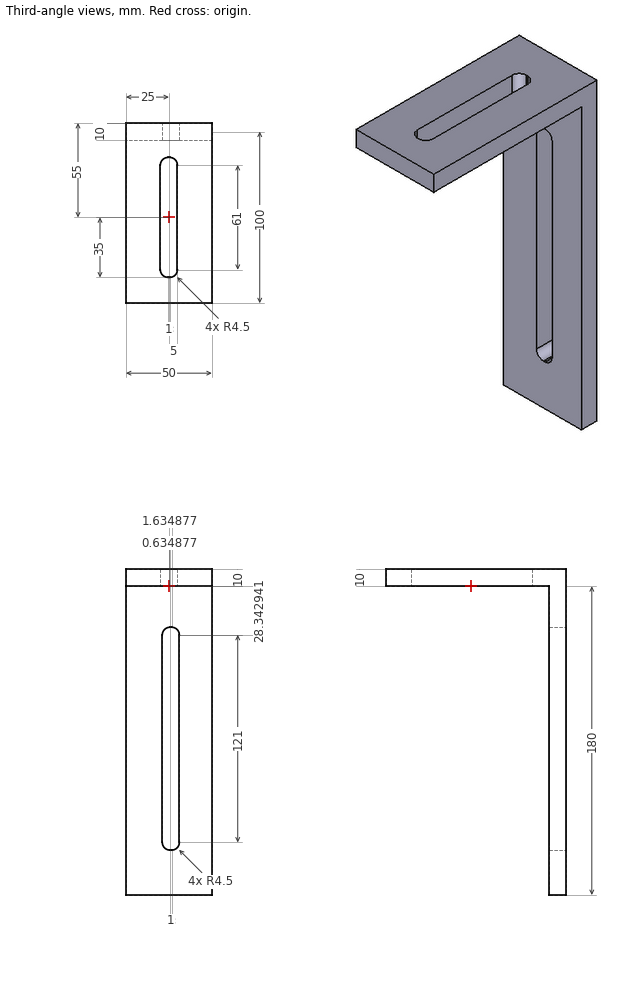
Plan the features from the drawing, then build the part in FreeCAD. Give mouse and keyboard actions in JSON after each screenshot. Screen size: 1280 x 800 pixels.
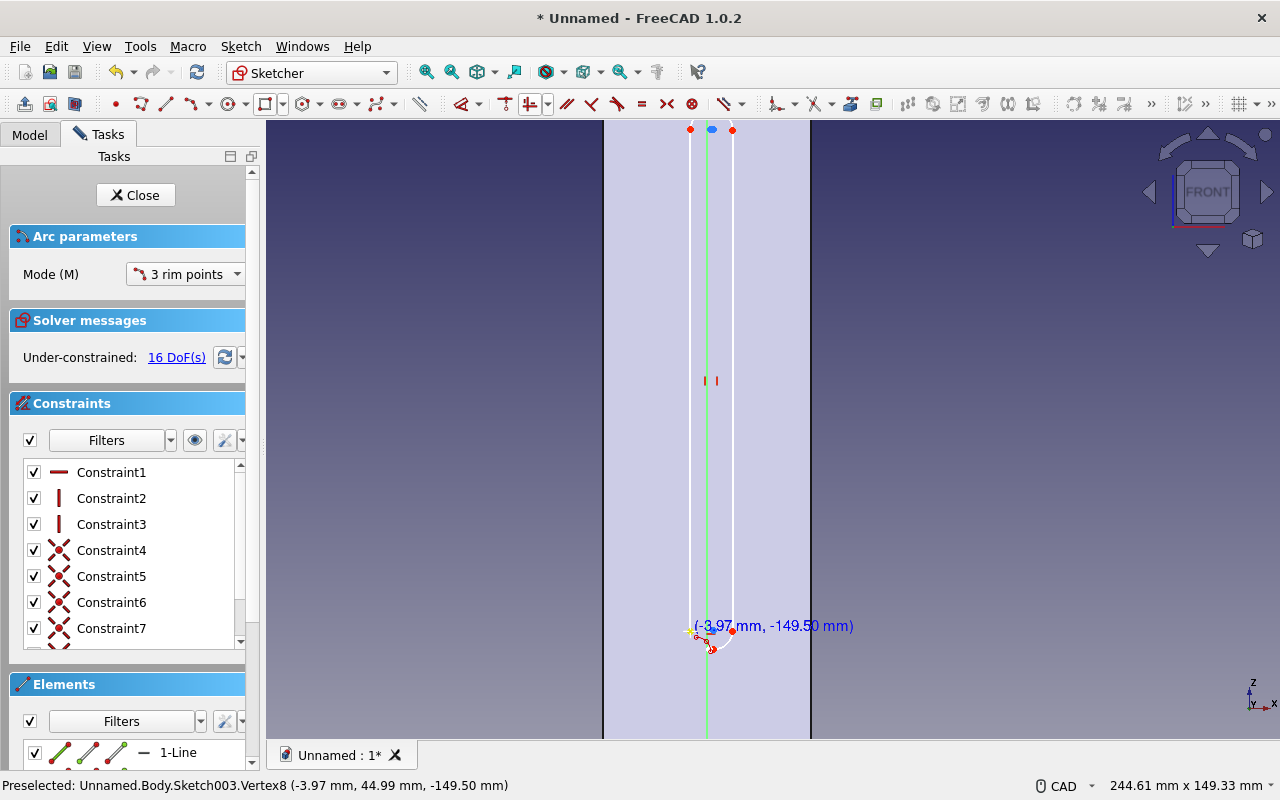
{"action": "scroll", "coordinate": [710, 649], "scroll_direction": "up", "scroll_amount": 11}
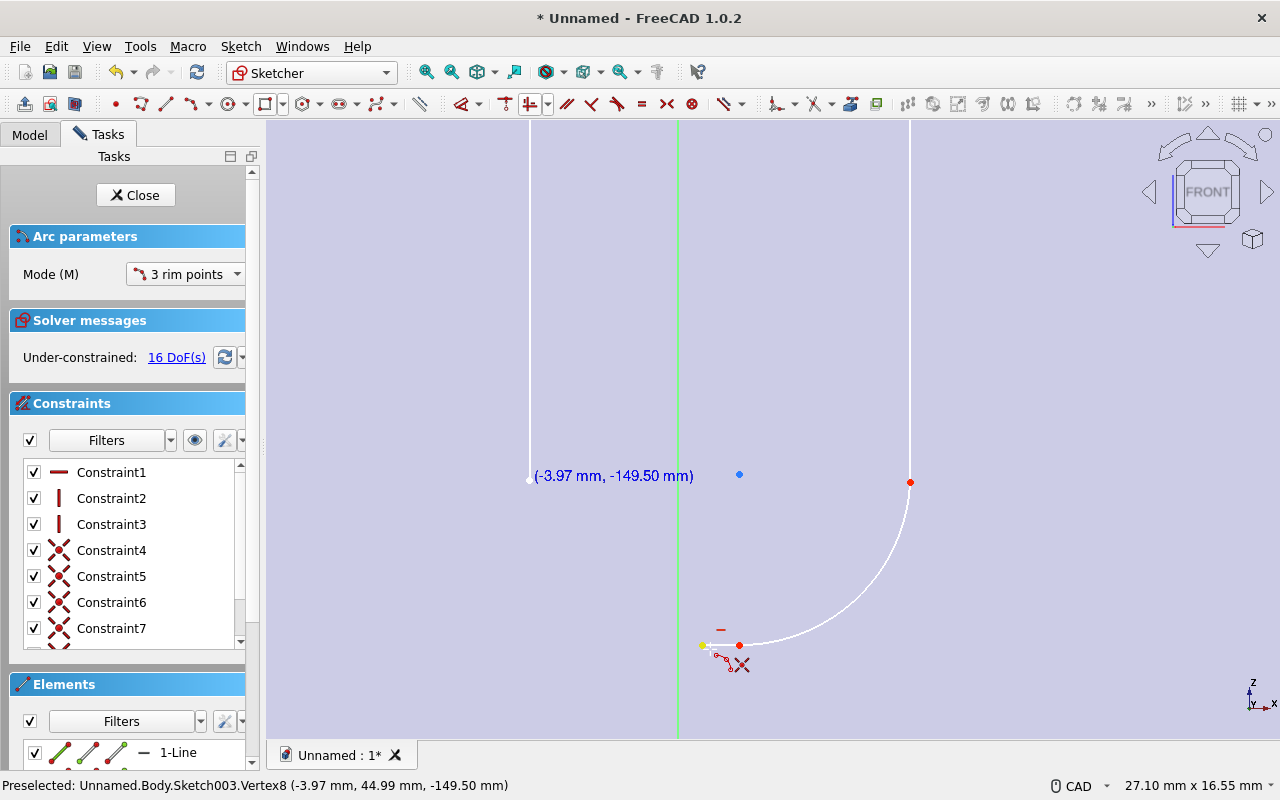
{"action": "left_click", "coordinate": [702, 645]}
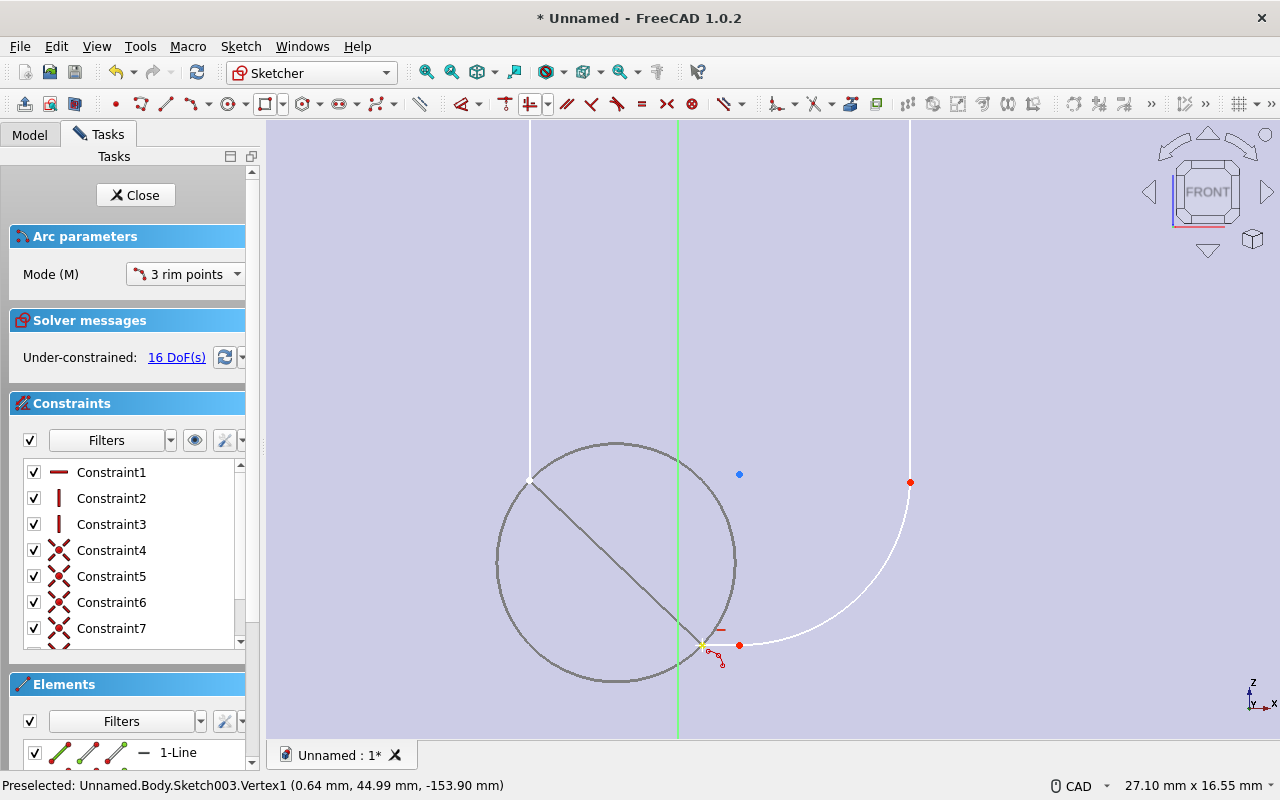
{"action": "scroll", "coordinate": [703, 643], "scroll_direction": "down", "scroll_amount": 13}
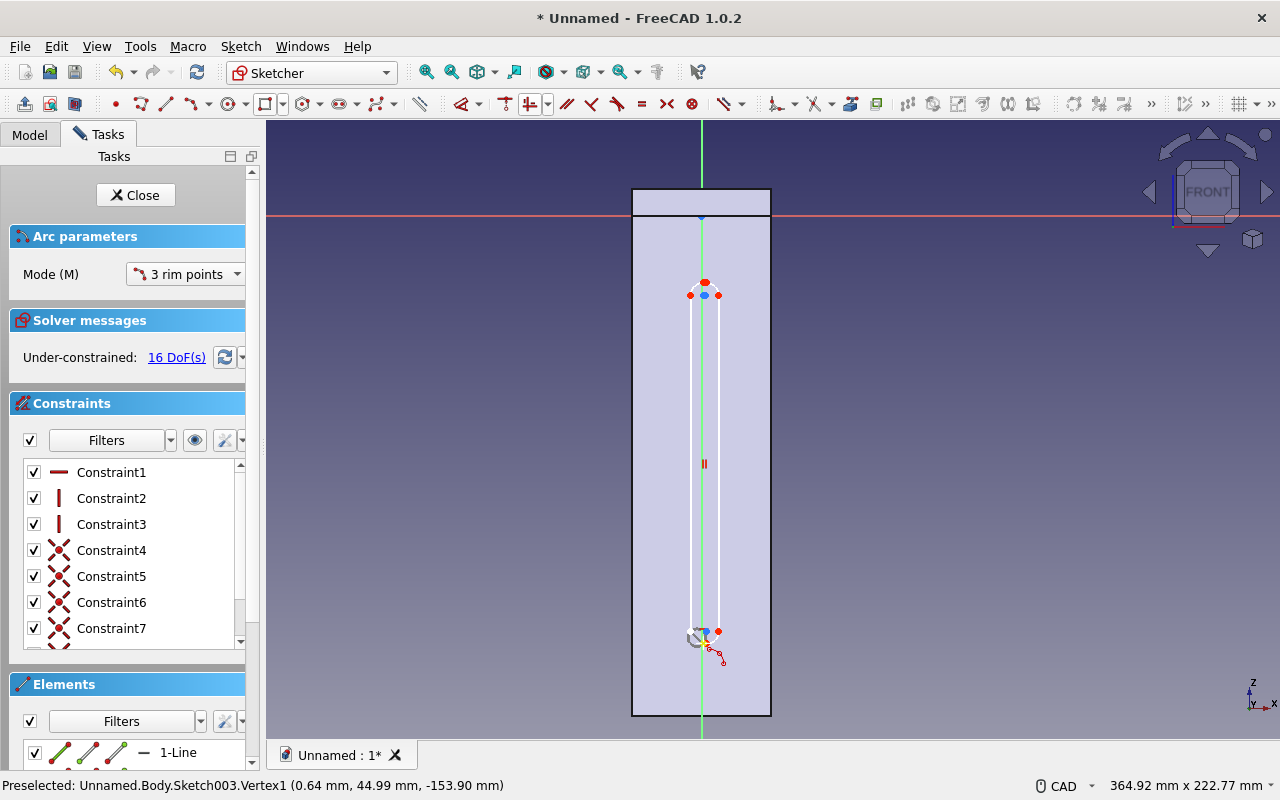
{"action": "scroll", "coordinate": [694, 640], "scroll_direction": "up", "scroll_amount": 8}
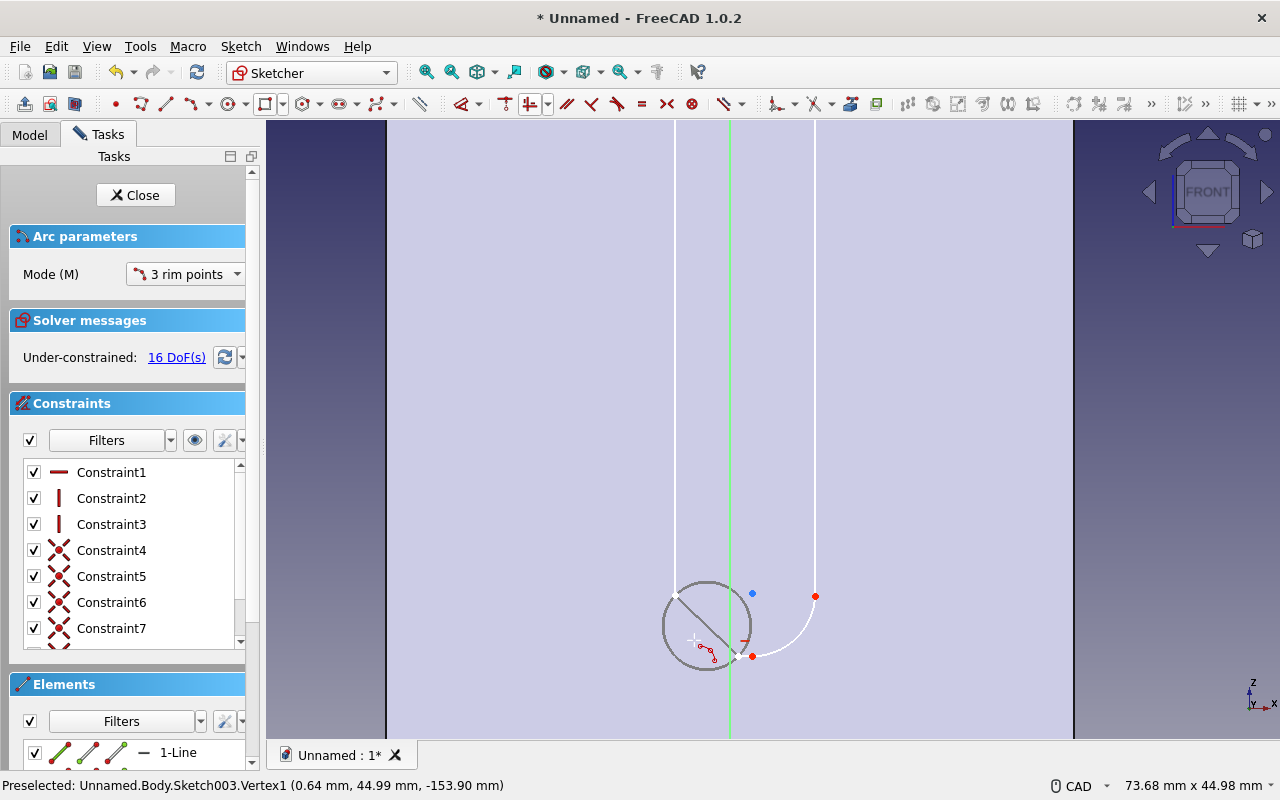
{"action": "left_click", "coordinate": [695, 637]}
{"action": "key", "text": "Escape"}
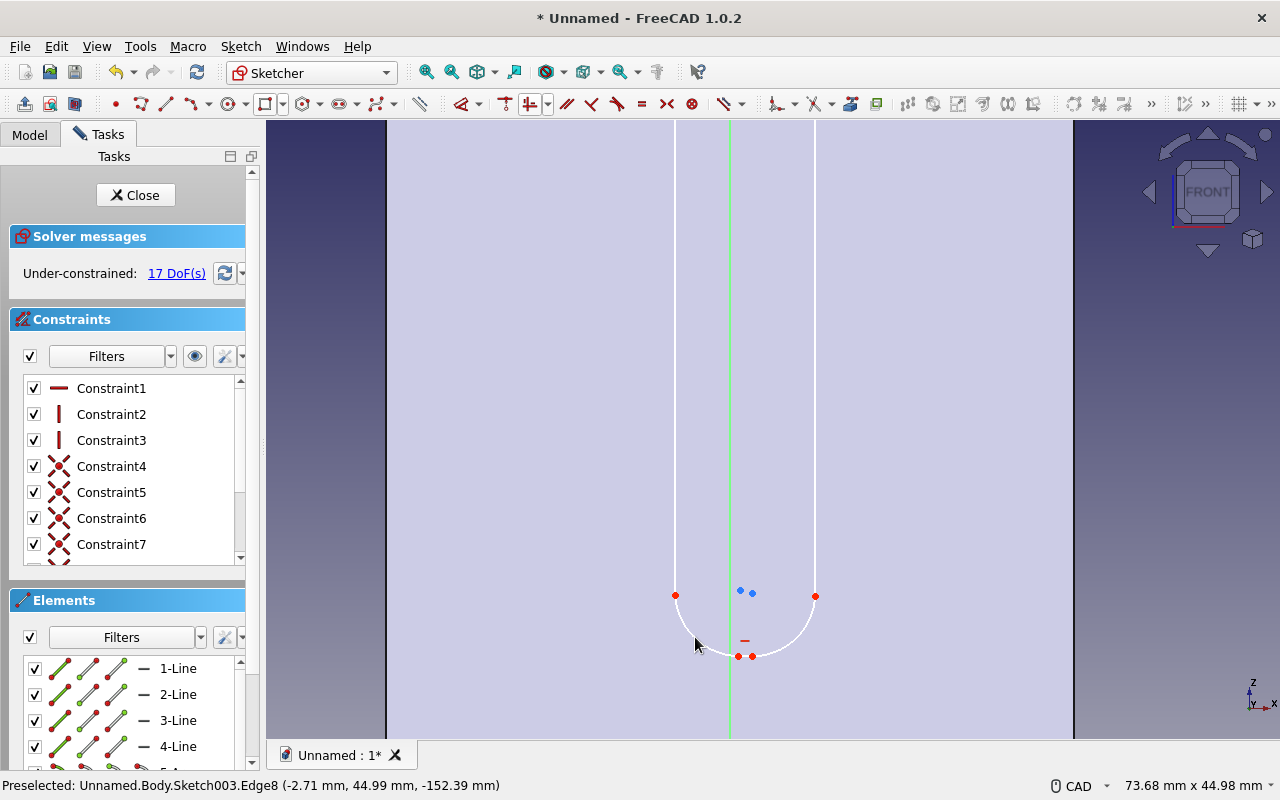
{"action": "scroll", "coordinate": [746, 656], "scroll_direction": "up", "scroll_amount": 4}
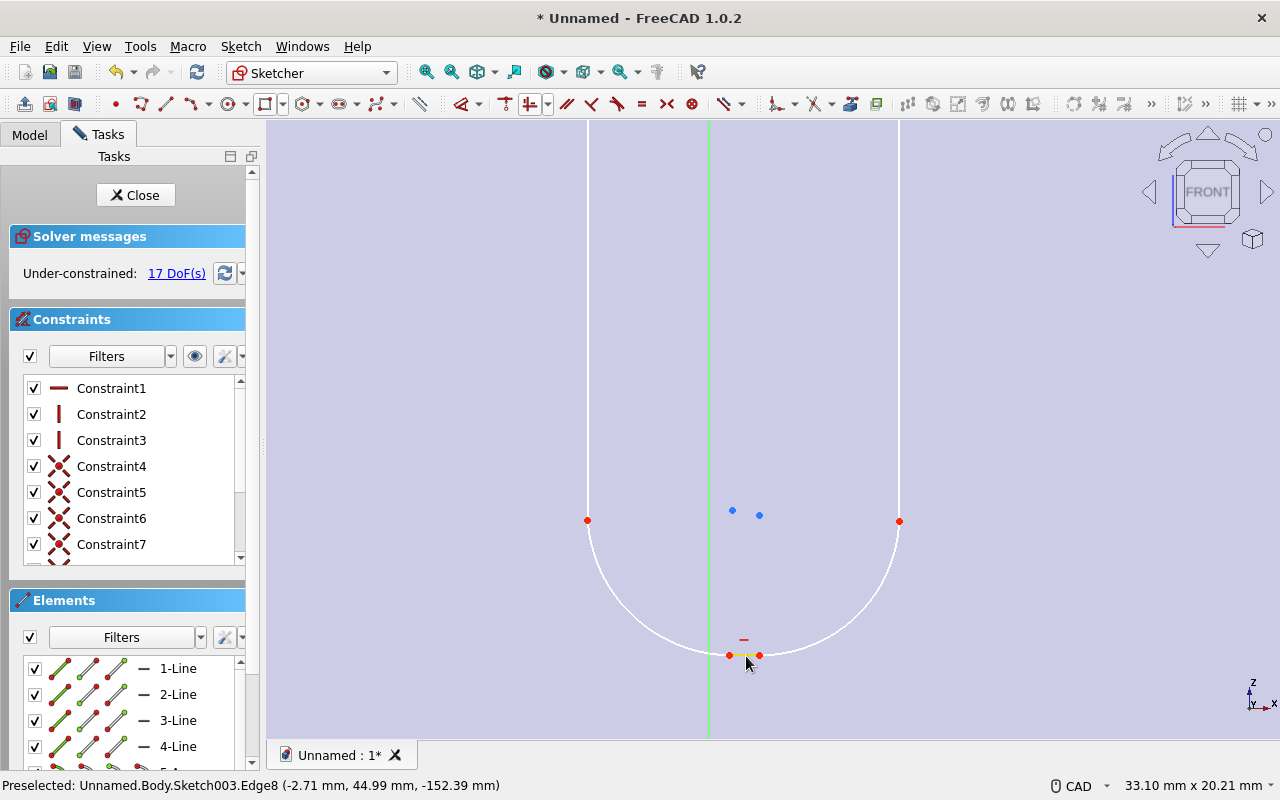
{"action": "left_click", "coordinate": [744, 655]}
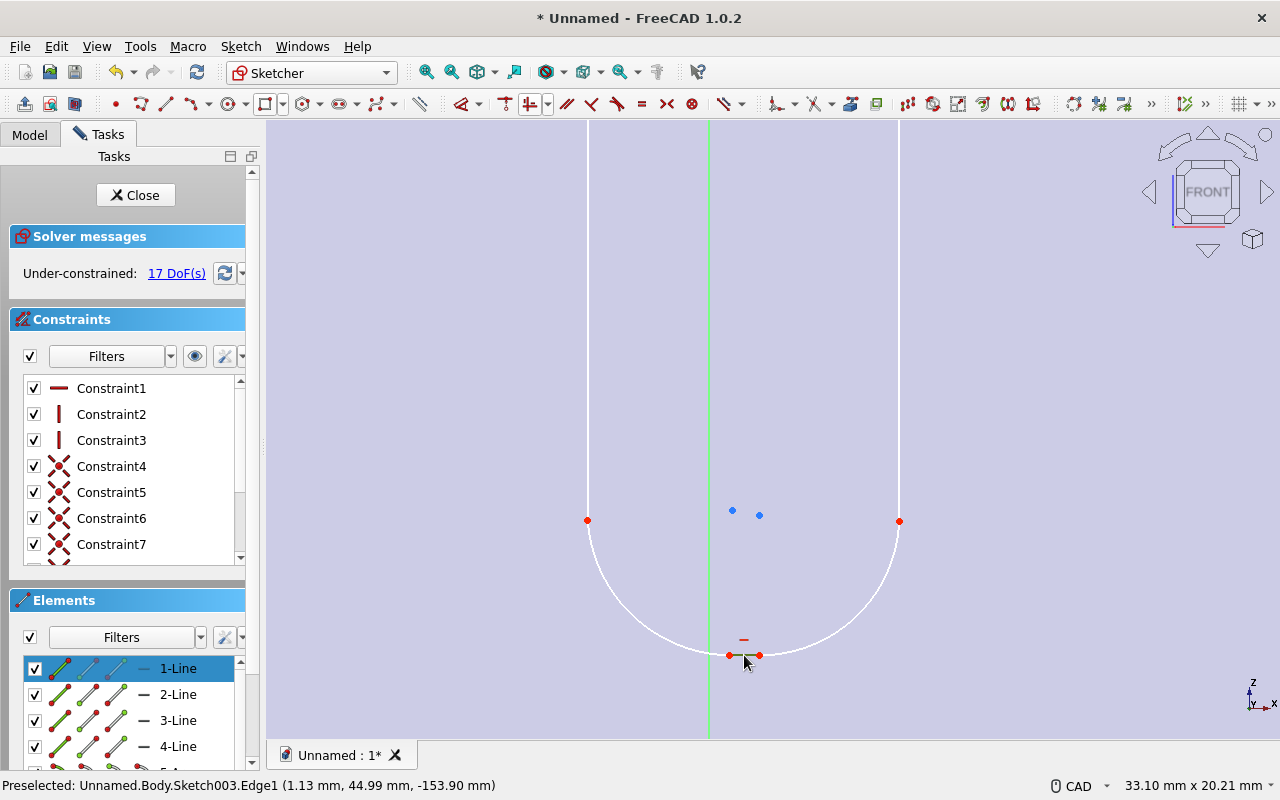
{"action": "scroll", "coordinate": [701, 642], "scroll_direction": "down", "scroll_amount": 12}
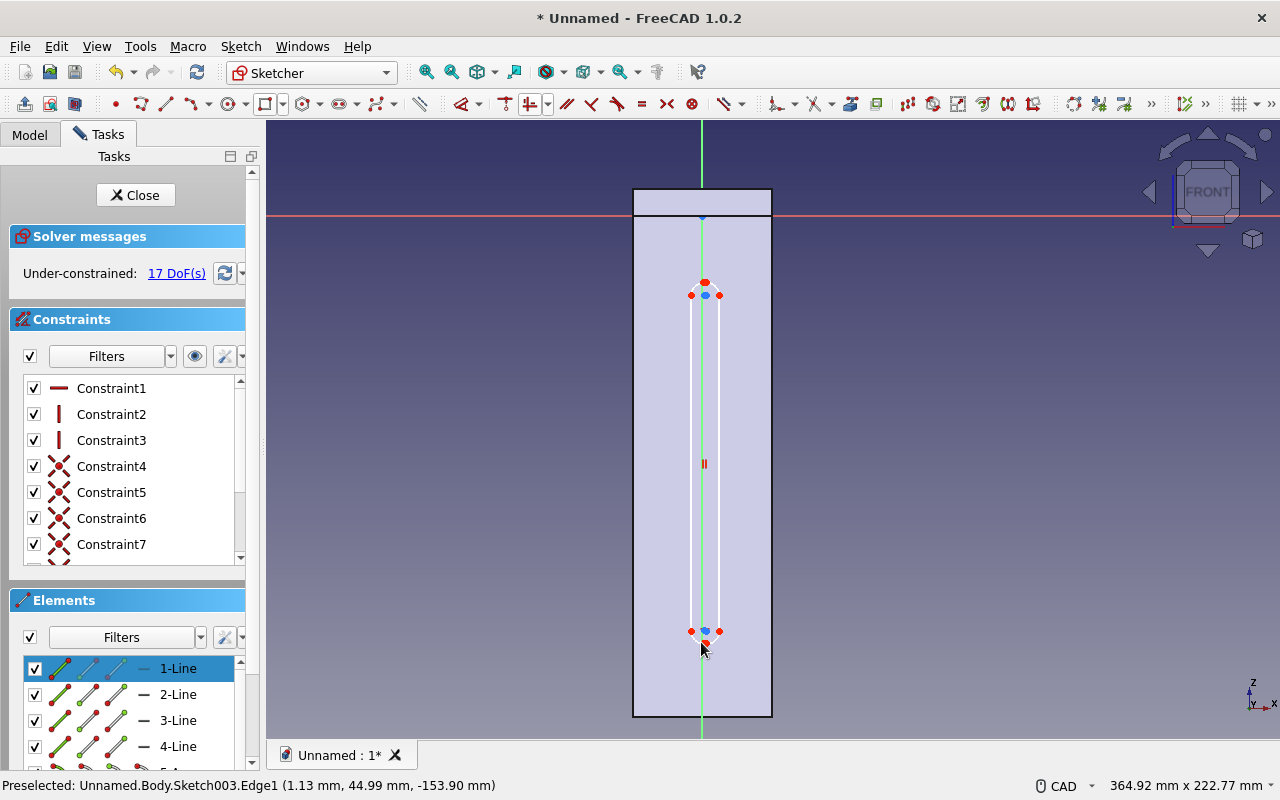
{"action": "scroll", "coordinate": [712, 643], "scroll_direction": "up", "scroll_amount": 5}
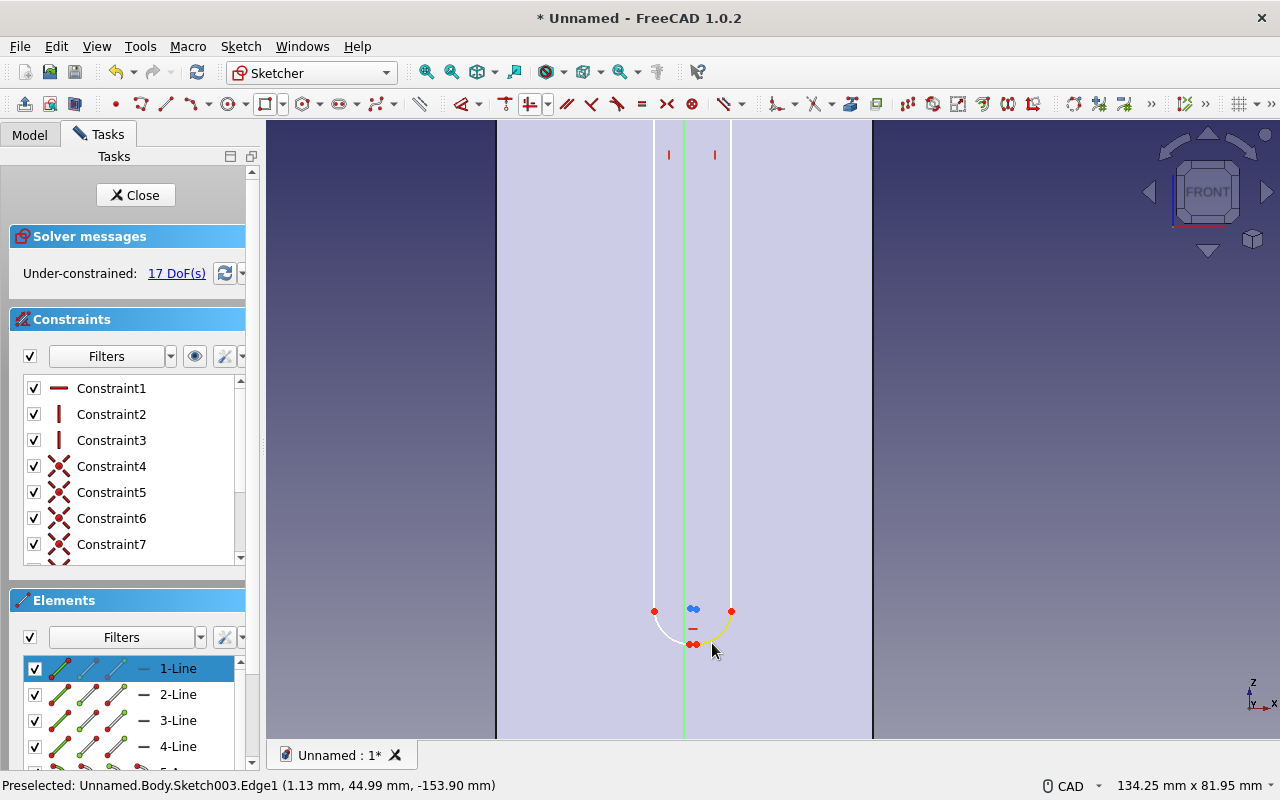
{"action": "left_click", "coordinate": [712, 641]}